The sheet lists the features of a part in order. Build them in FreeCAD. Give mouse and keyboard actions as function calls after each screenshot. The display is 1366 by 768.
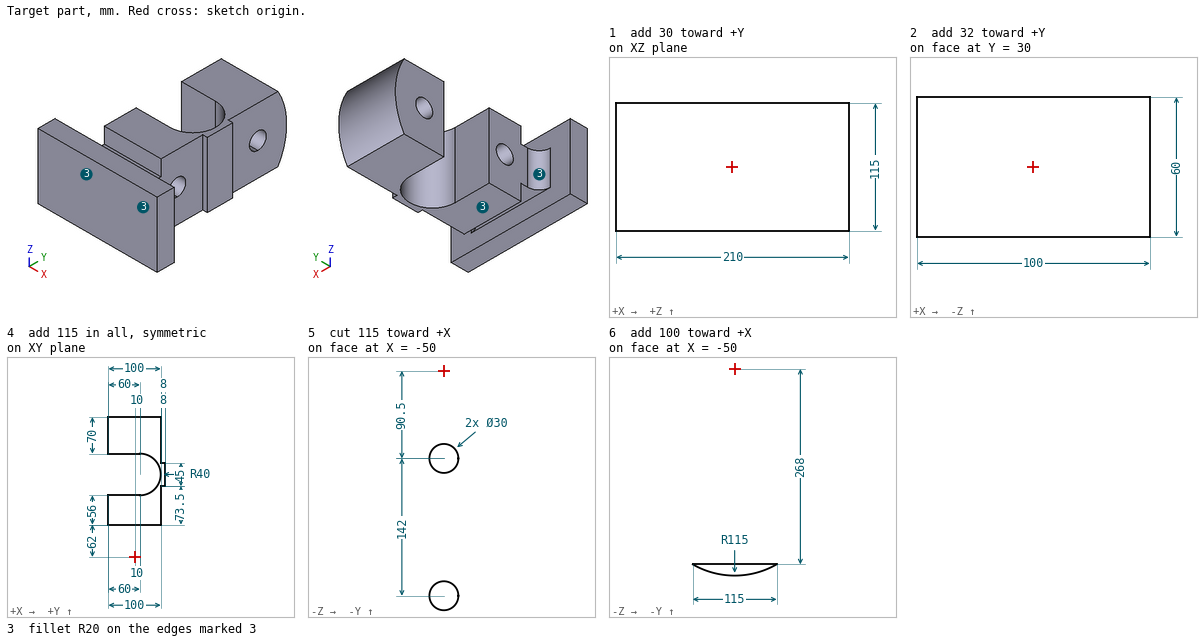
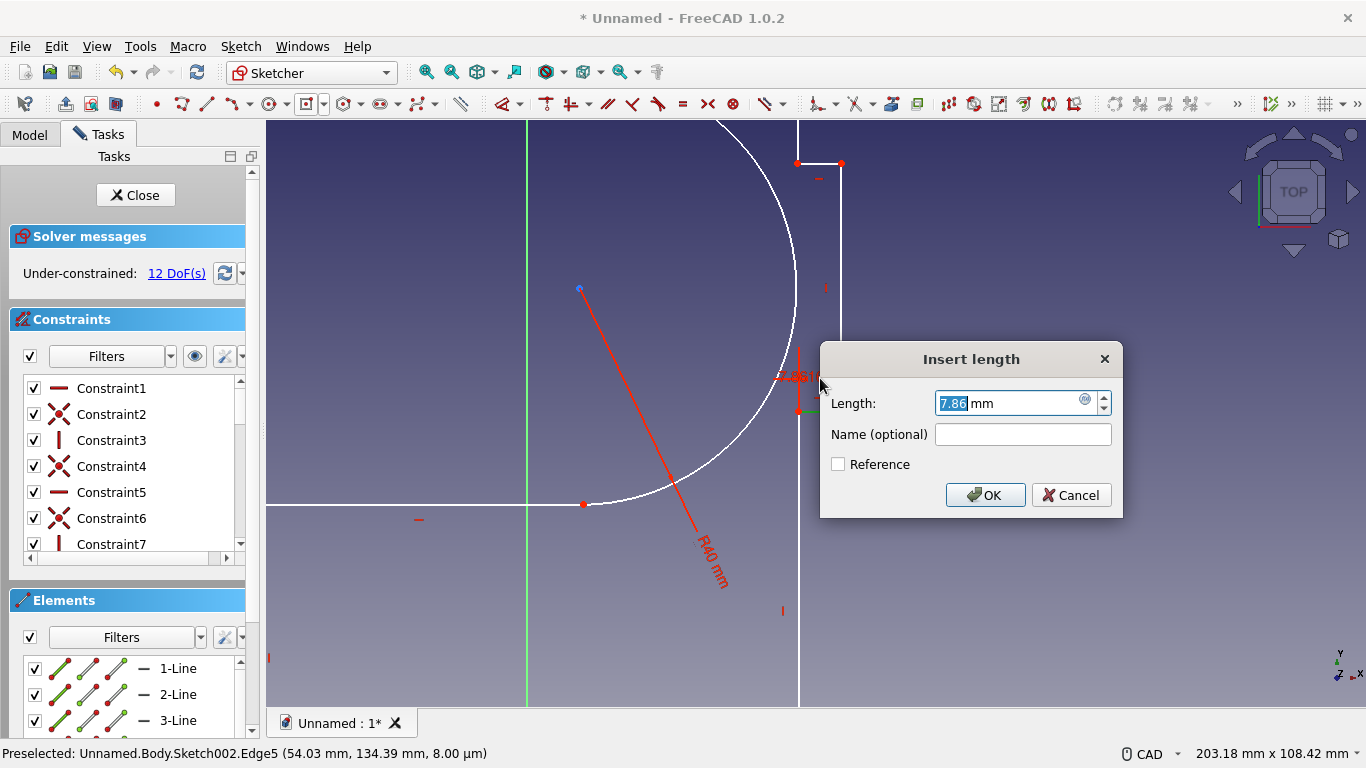
text(8)
key(Return)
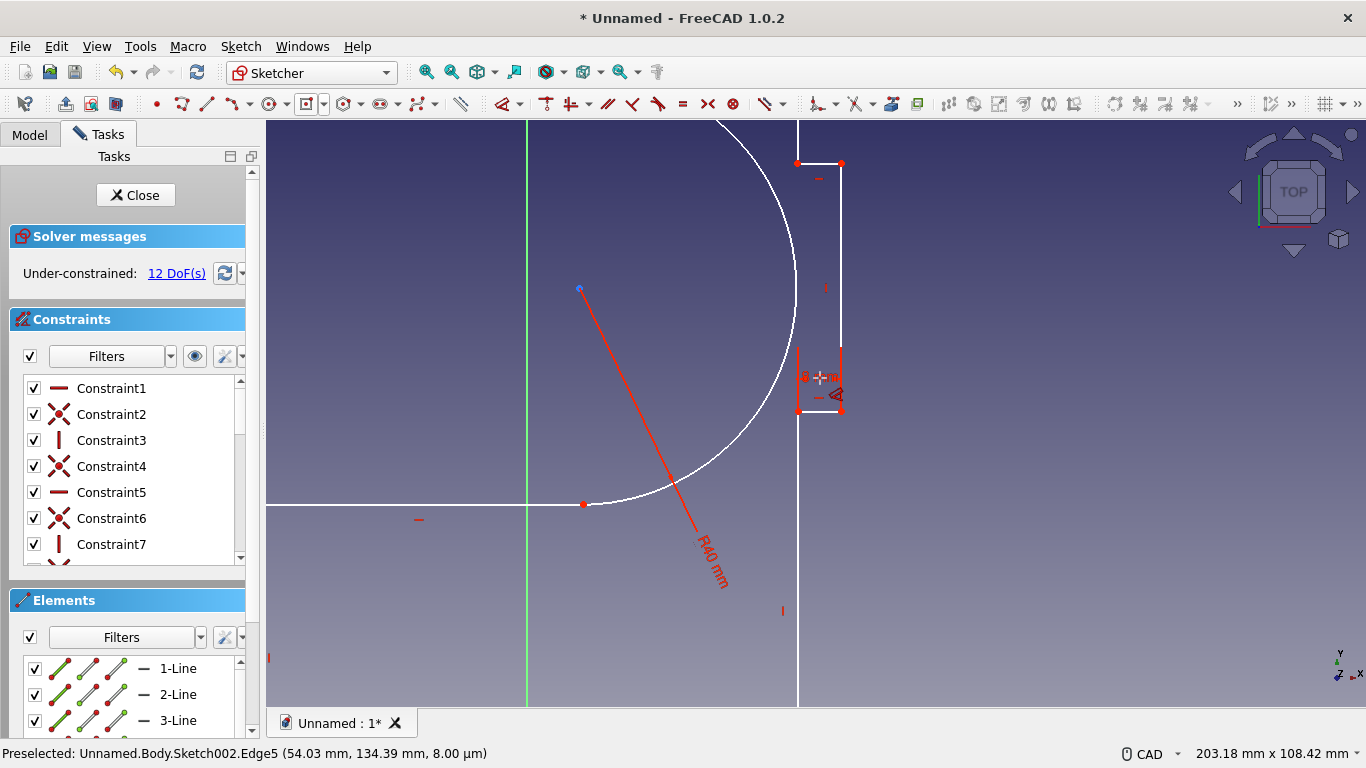
click(828, 164)
click(819, 198)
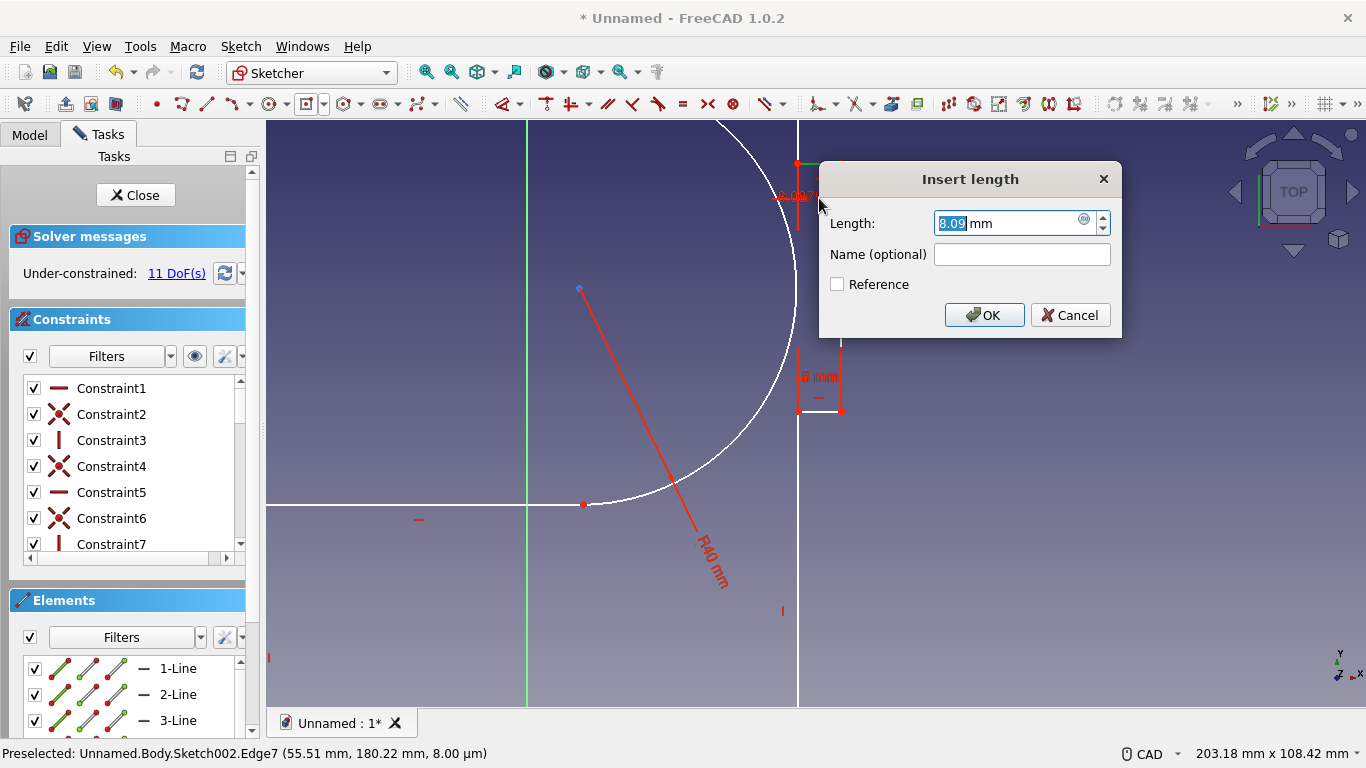
text(8)
key(Return)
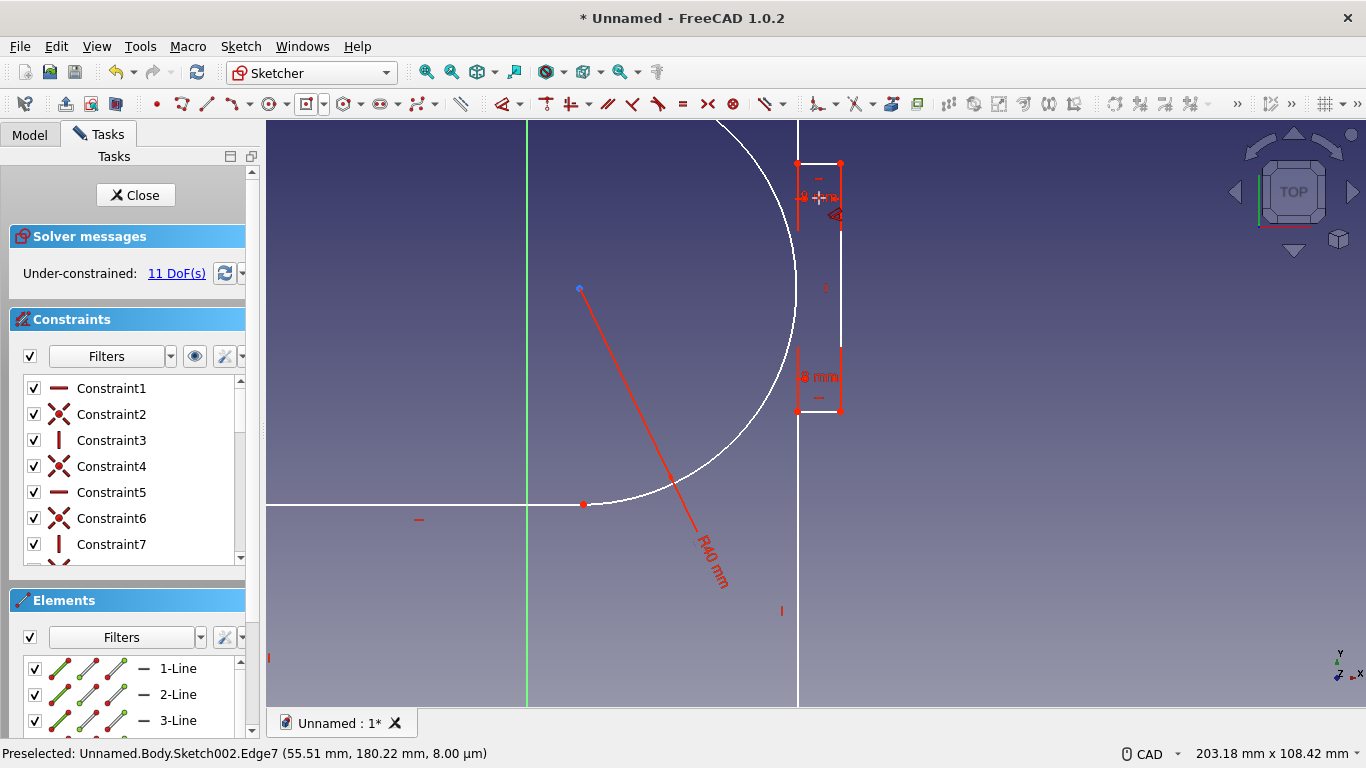
scroll(812, 413, down, 7)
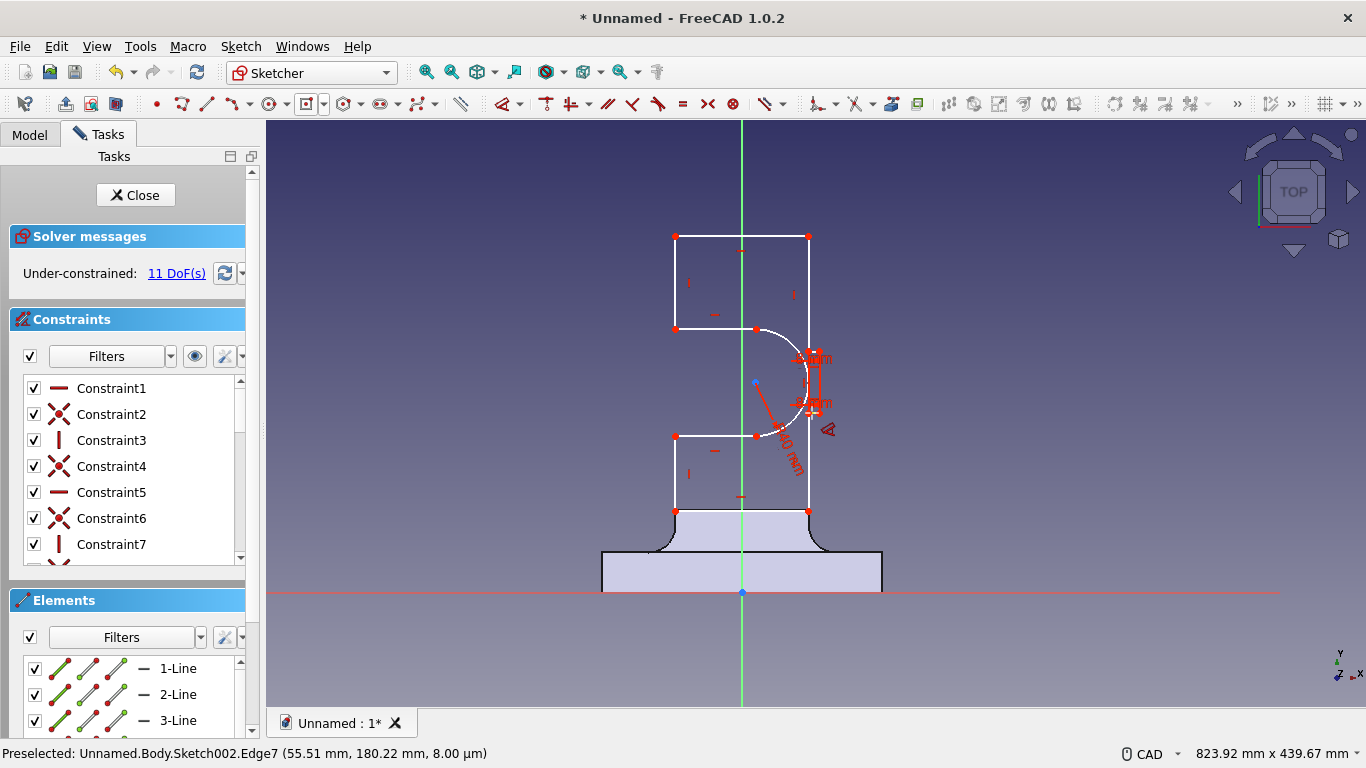
scroll(732, 436, up, 2)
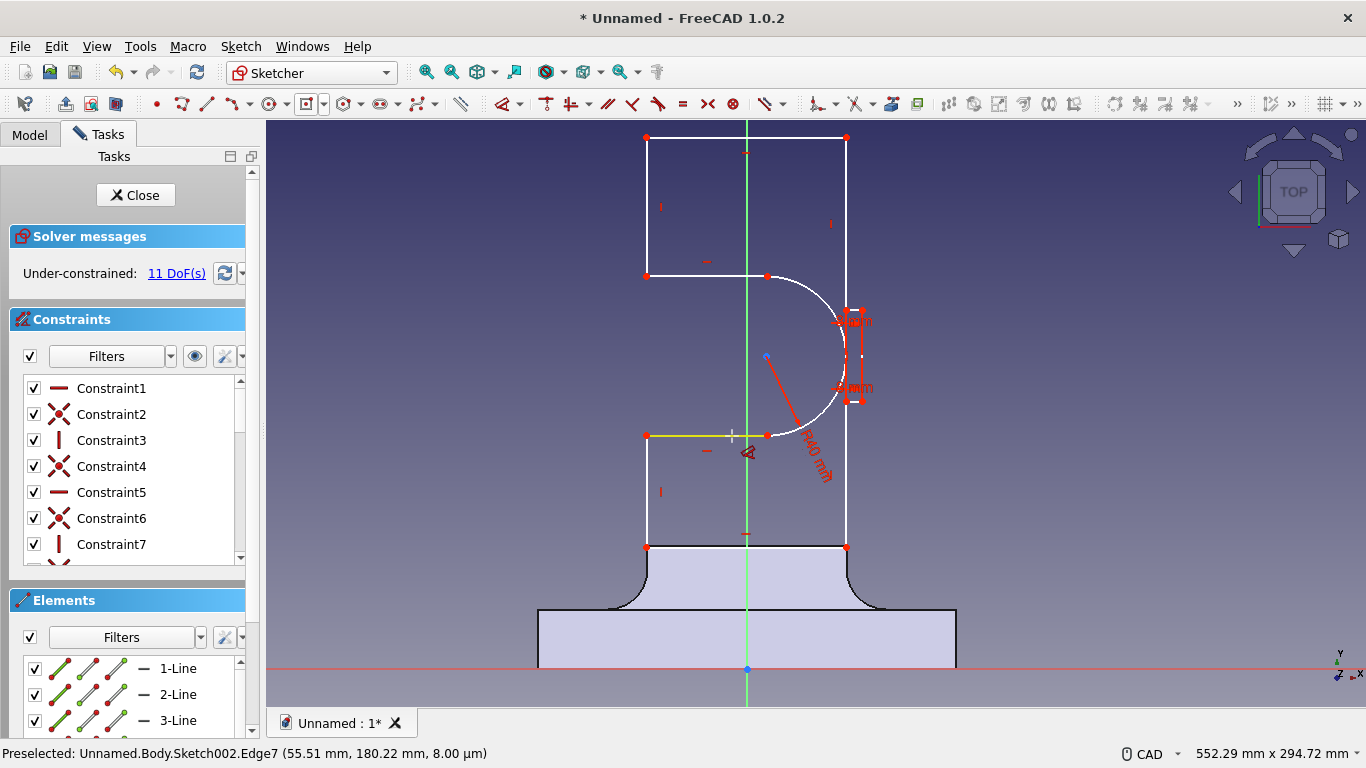
click(731, 436)
click(707, 470)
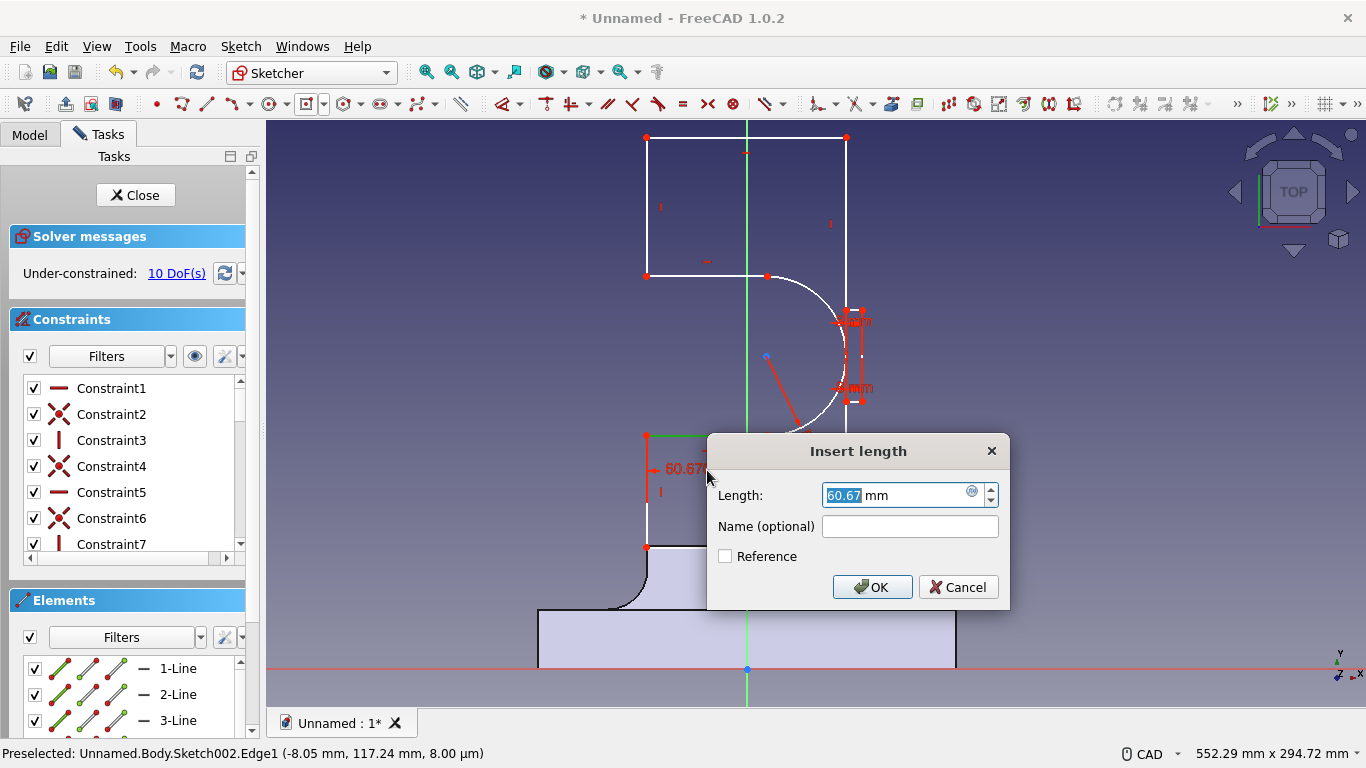
text(60)
key(Return)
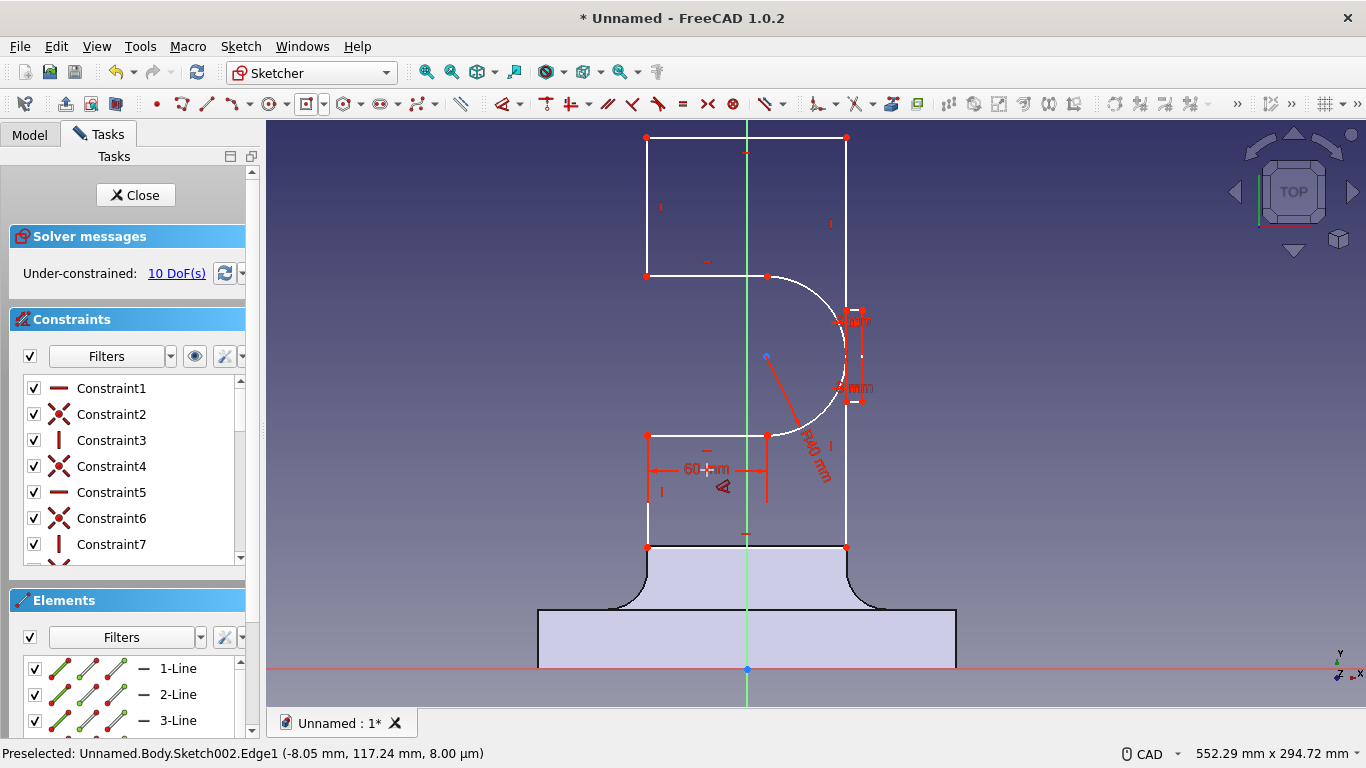
click(648, 469)
click(614, 492)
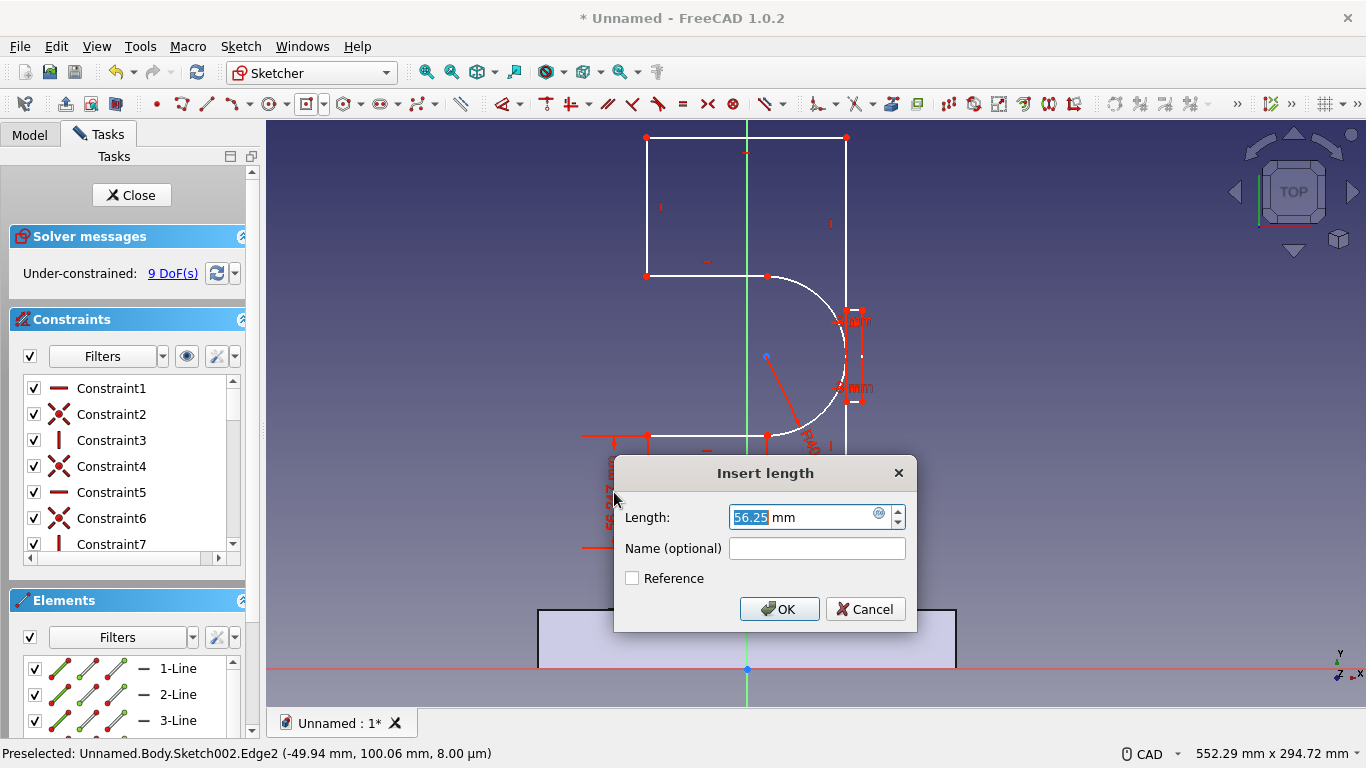
text(56)
key(Return)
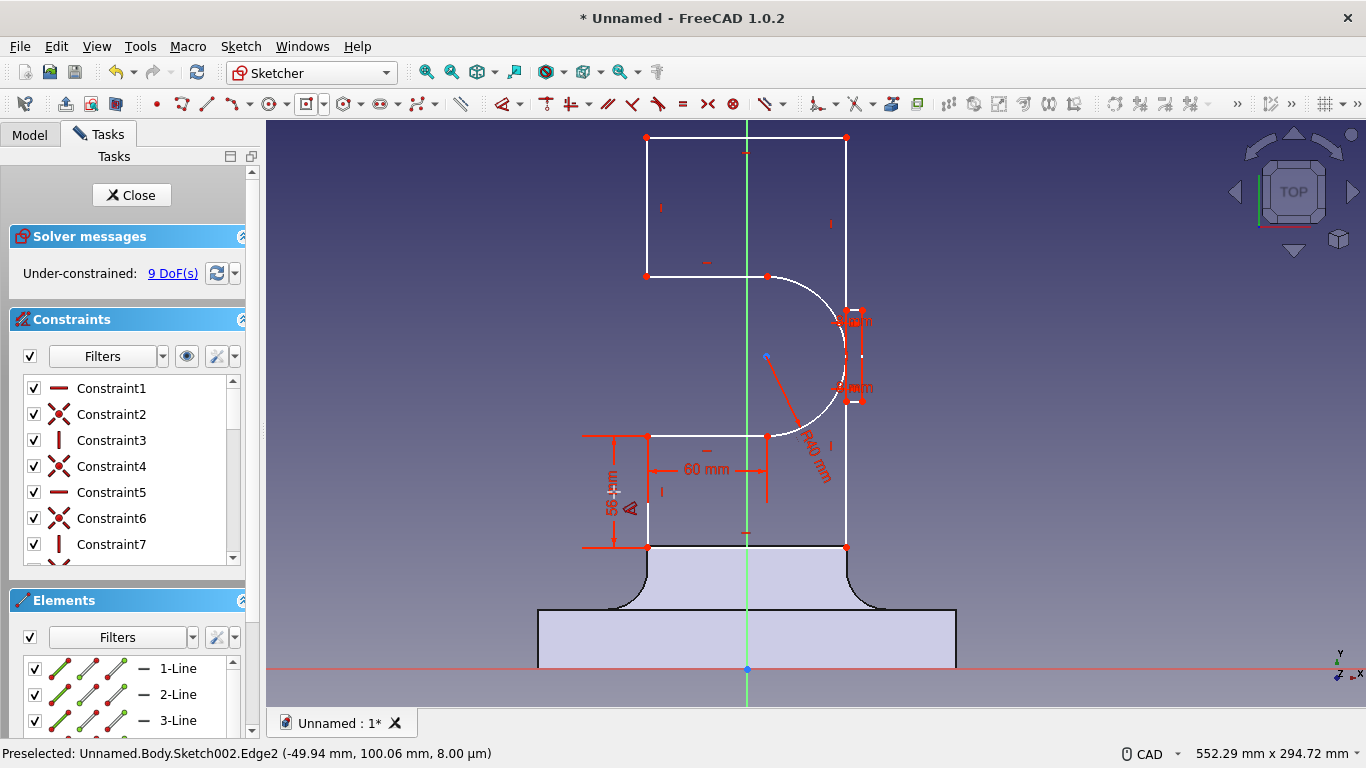
click(862, 374)
click(896, 356)